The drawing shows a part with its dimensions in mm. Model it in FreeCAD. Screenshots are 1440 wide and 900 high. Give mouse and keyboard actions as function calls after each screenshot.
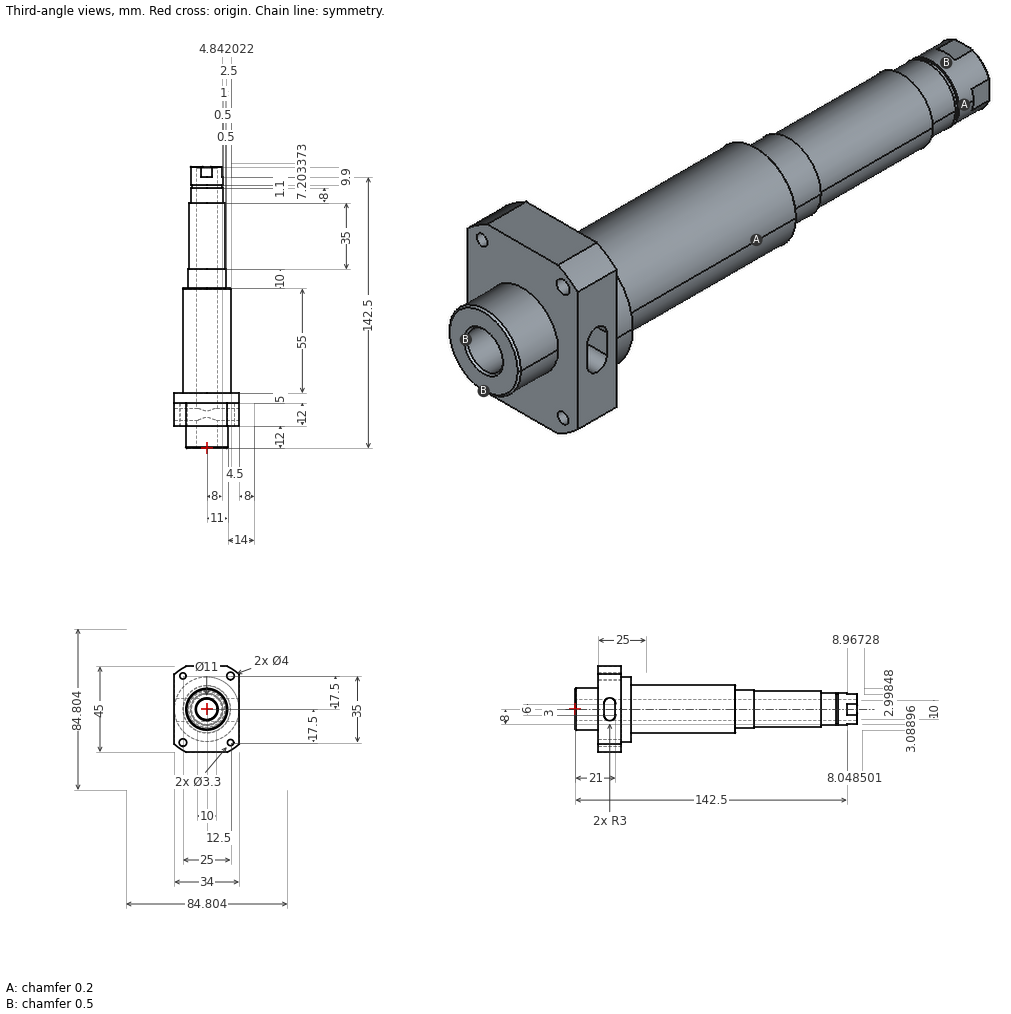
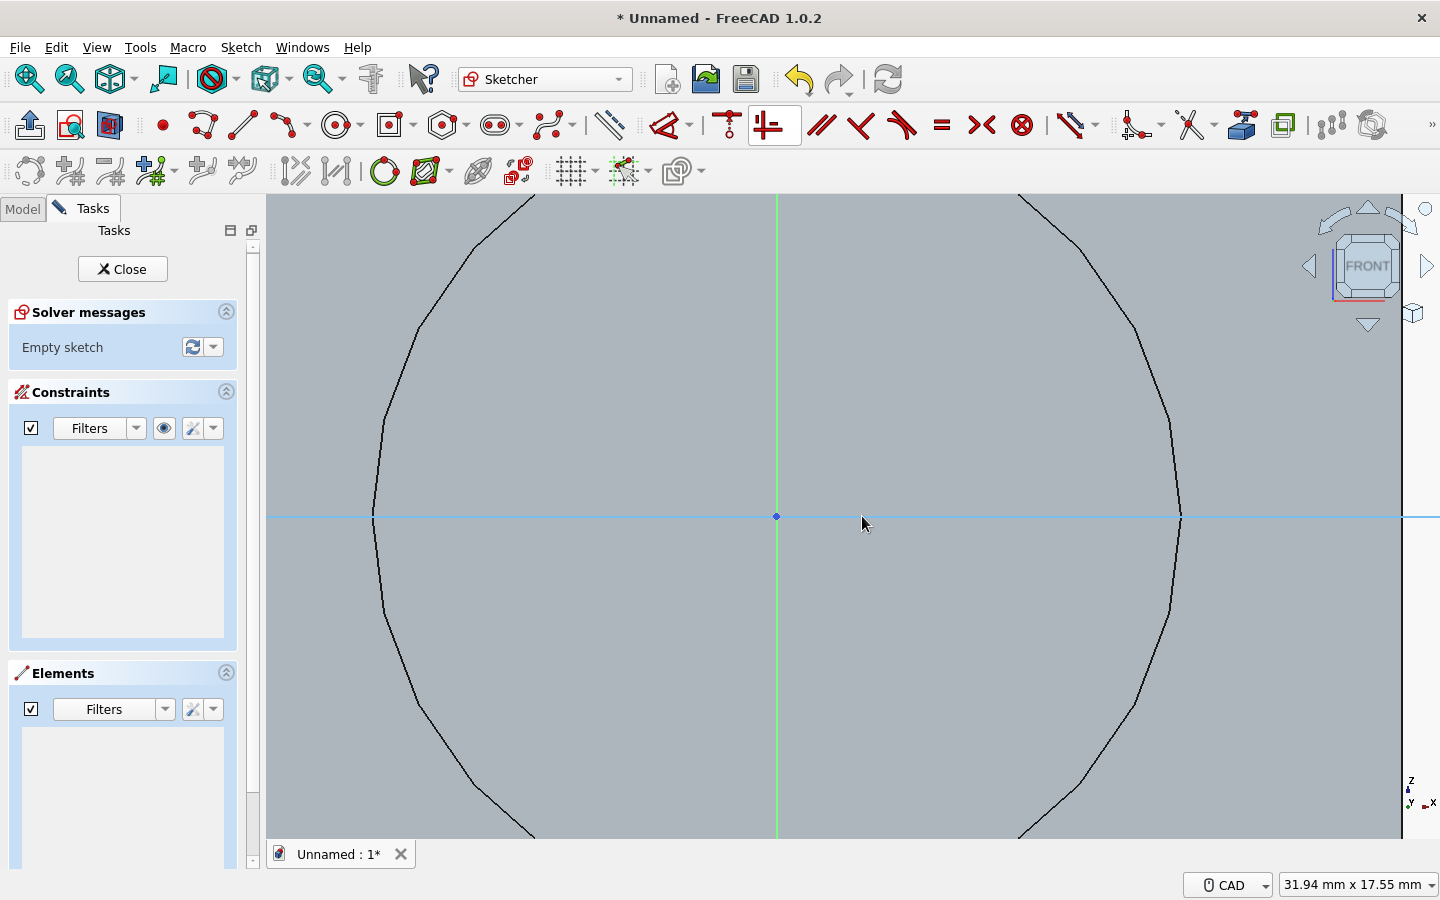
click(336, 126)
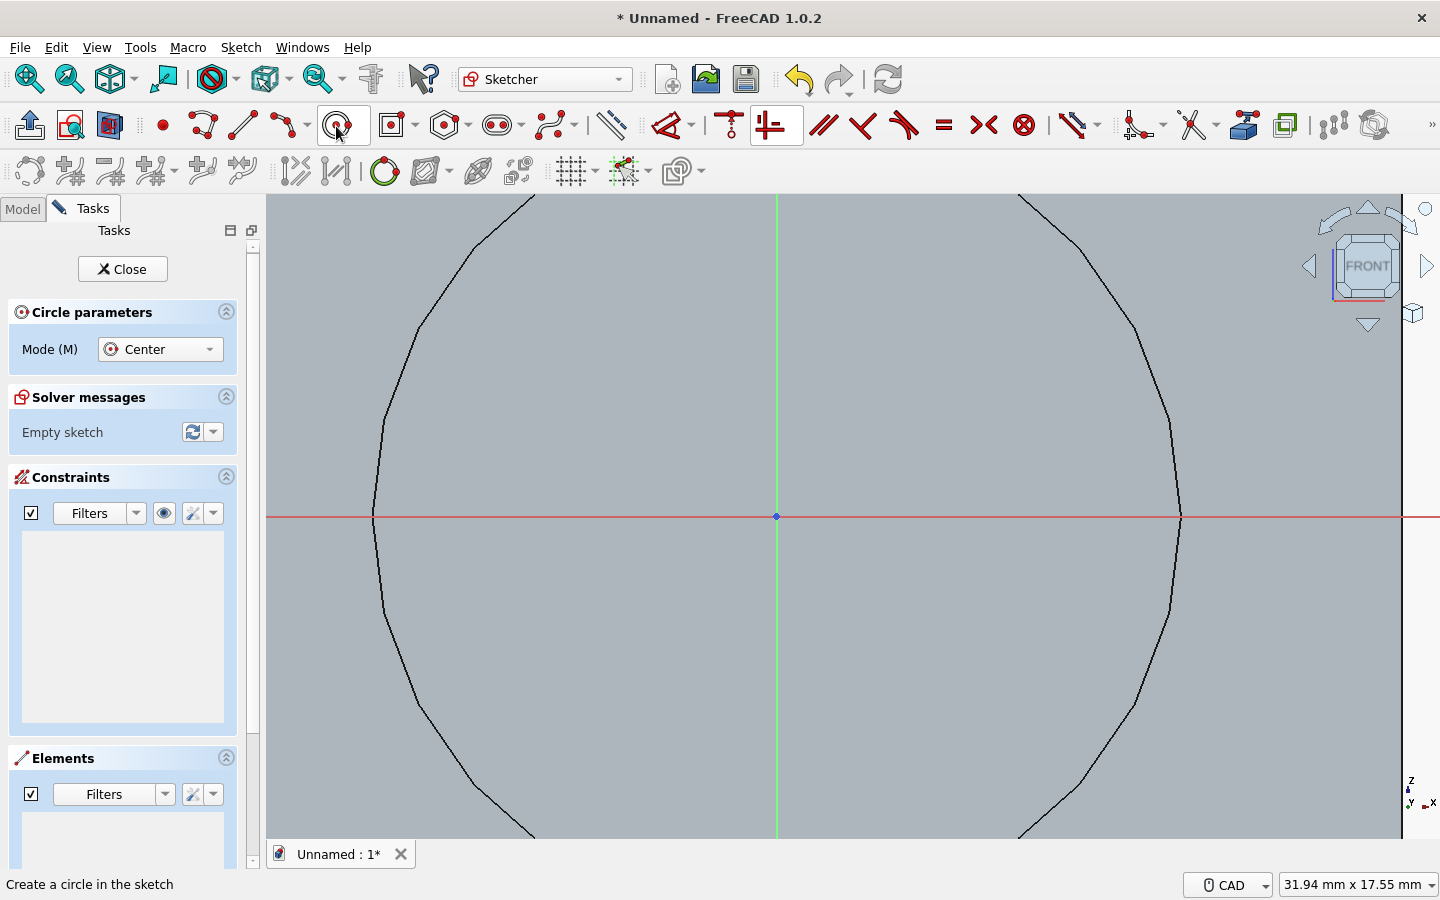
click(777, 516)
move(920, 374)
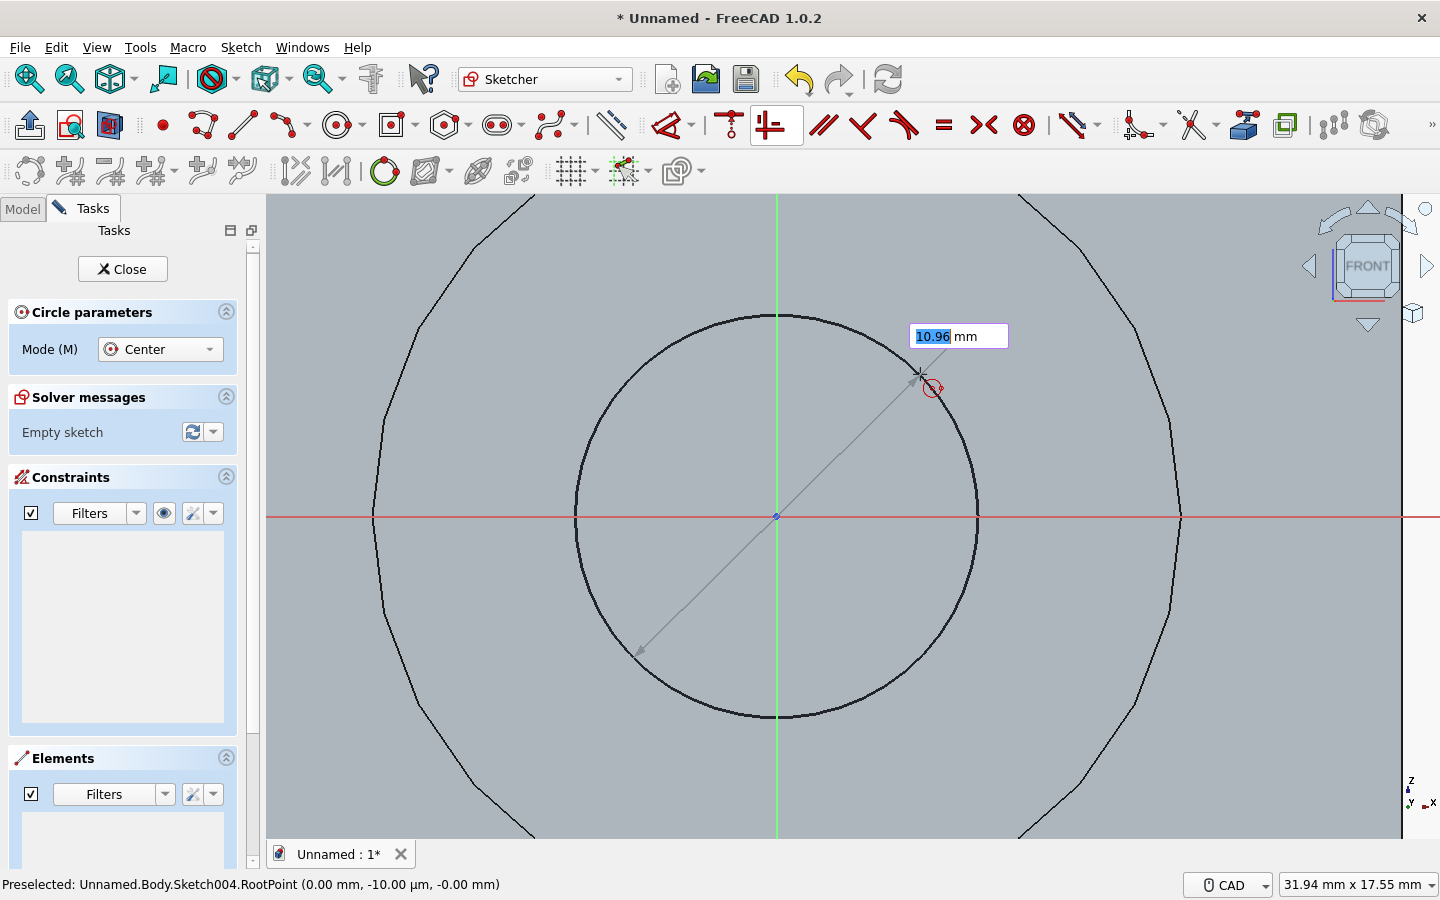
text(11)
key(Return)
key(Escape)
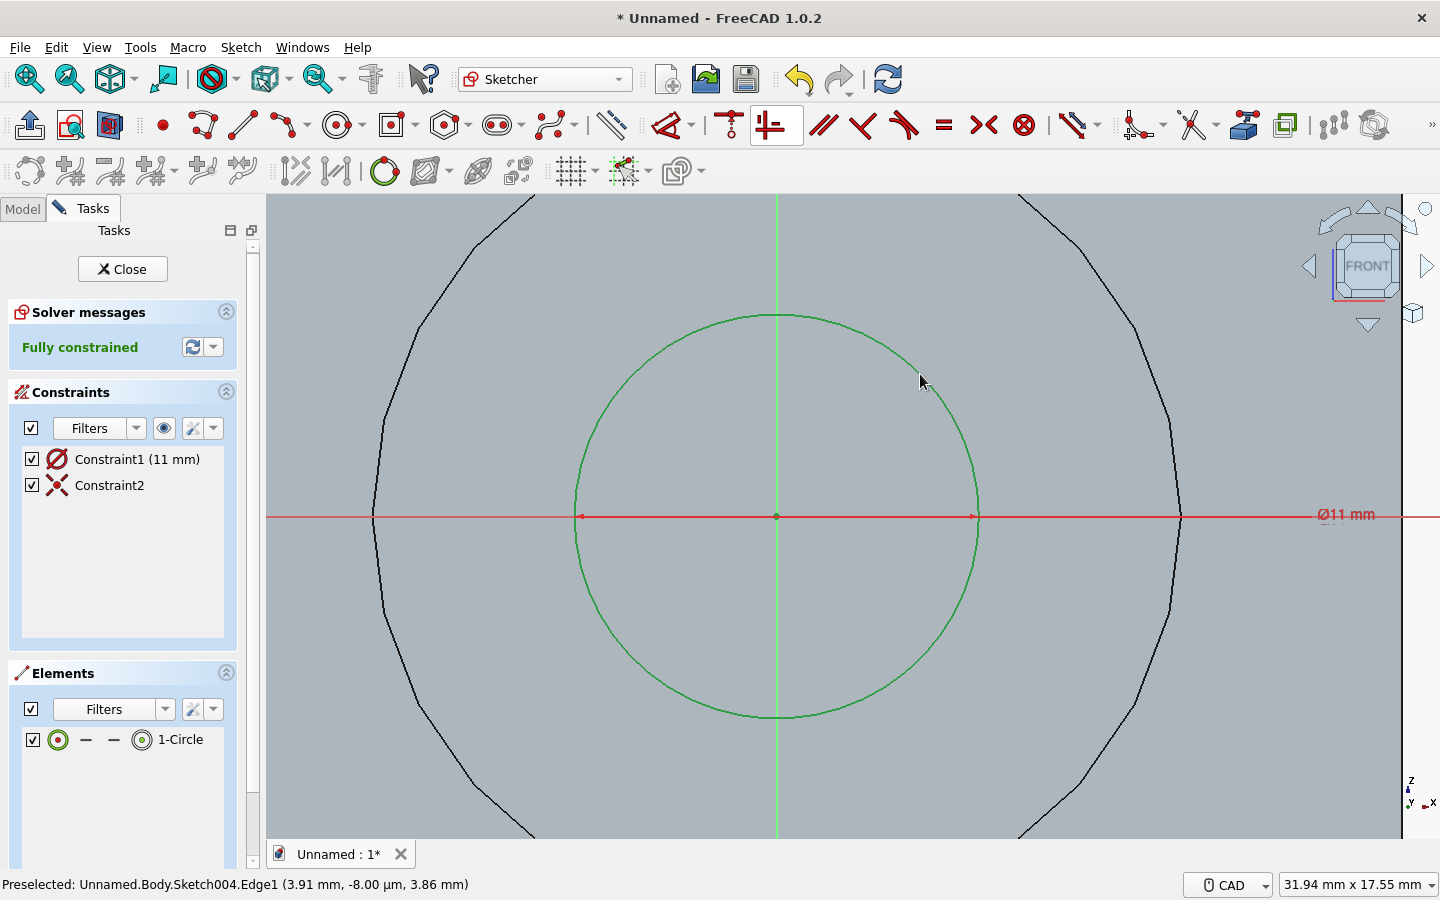
click(123, 269)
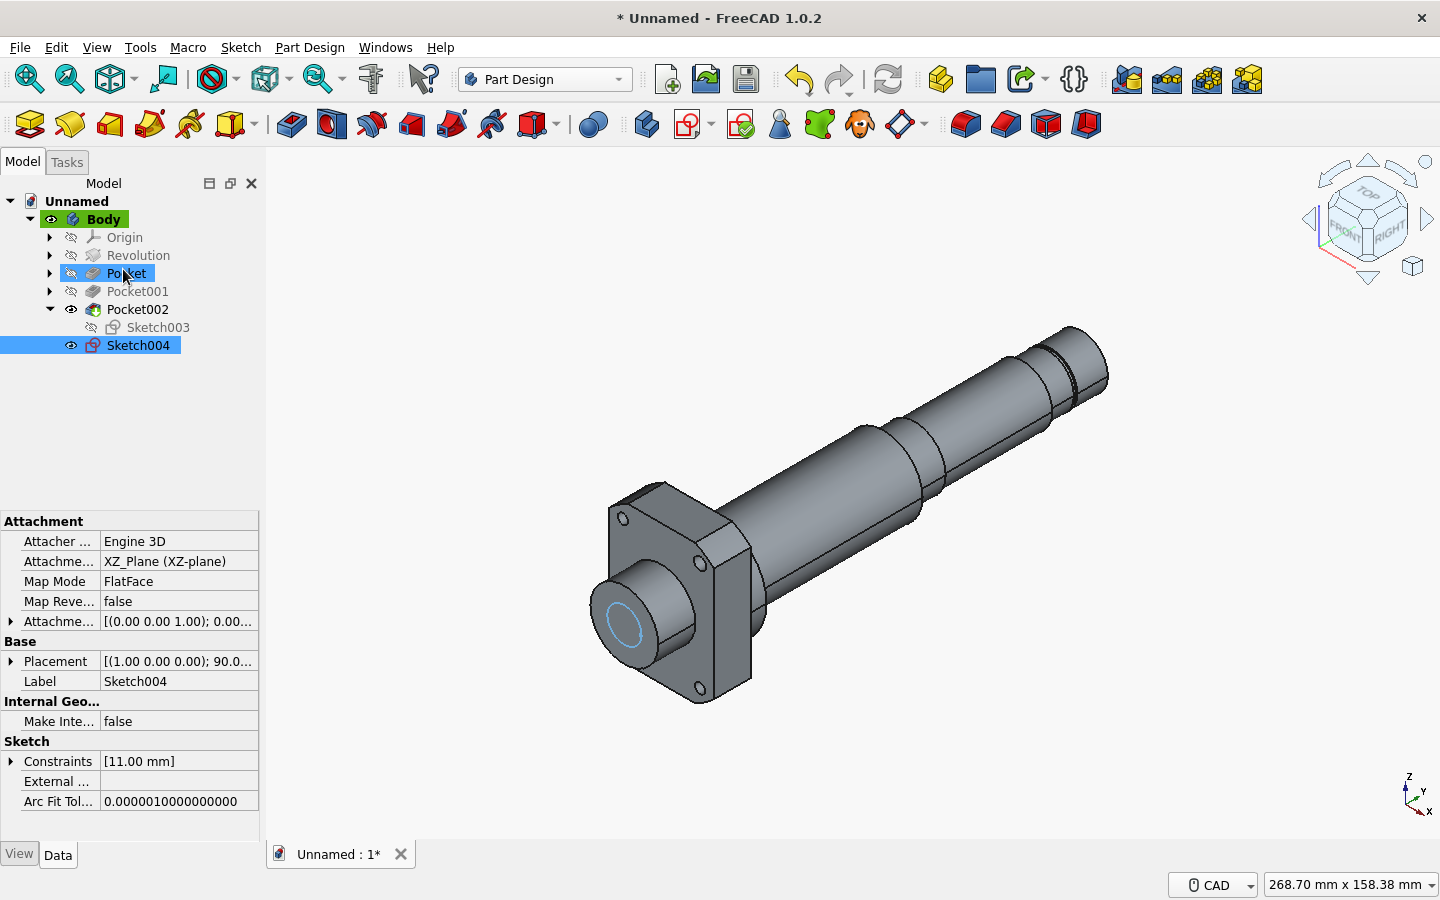
click(292, 124)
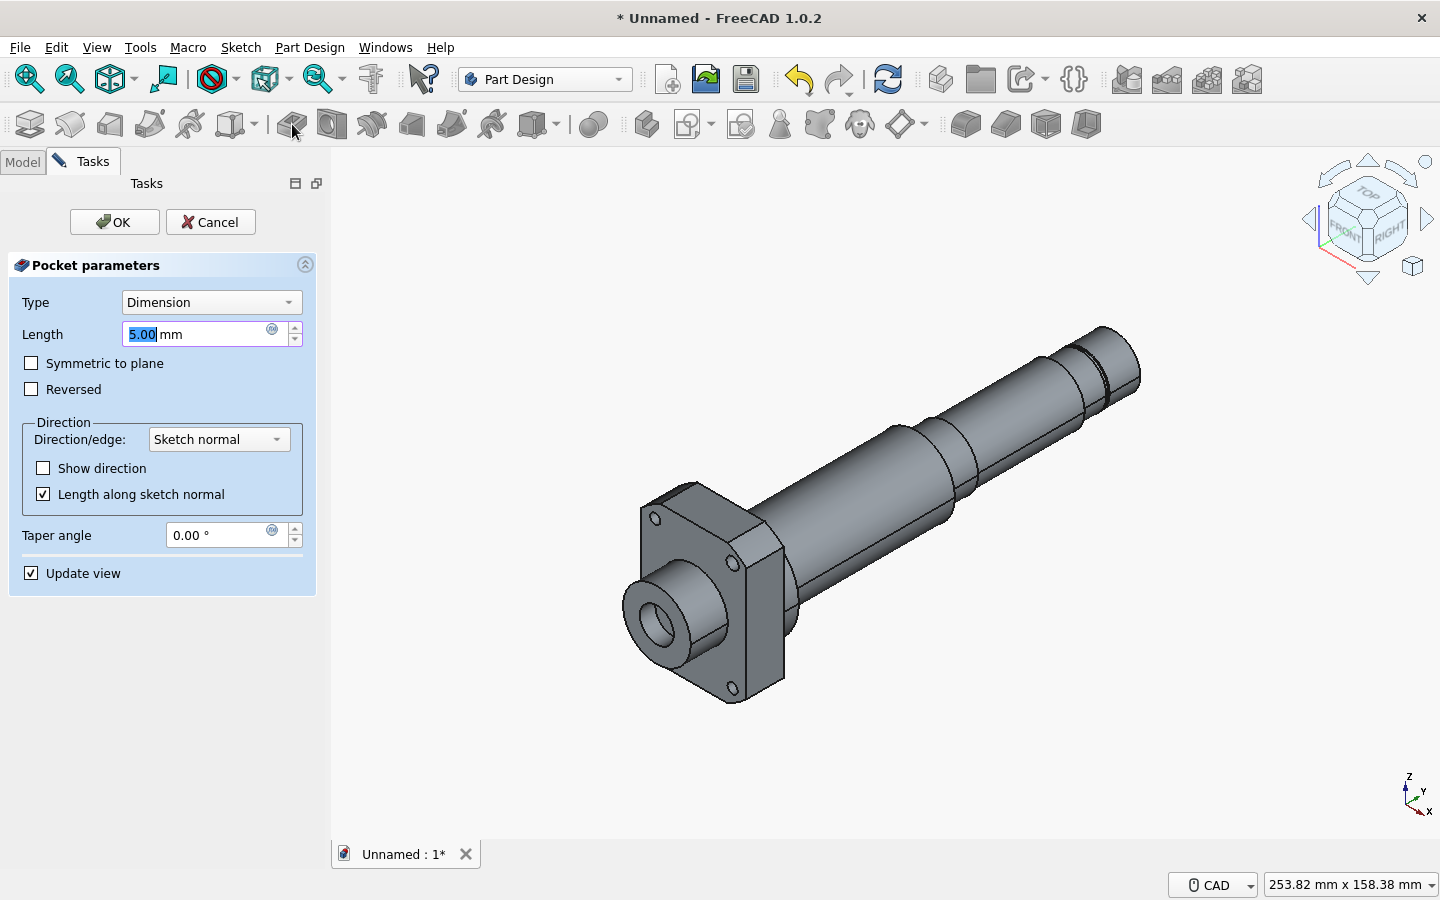
click(212, 302)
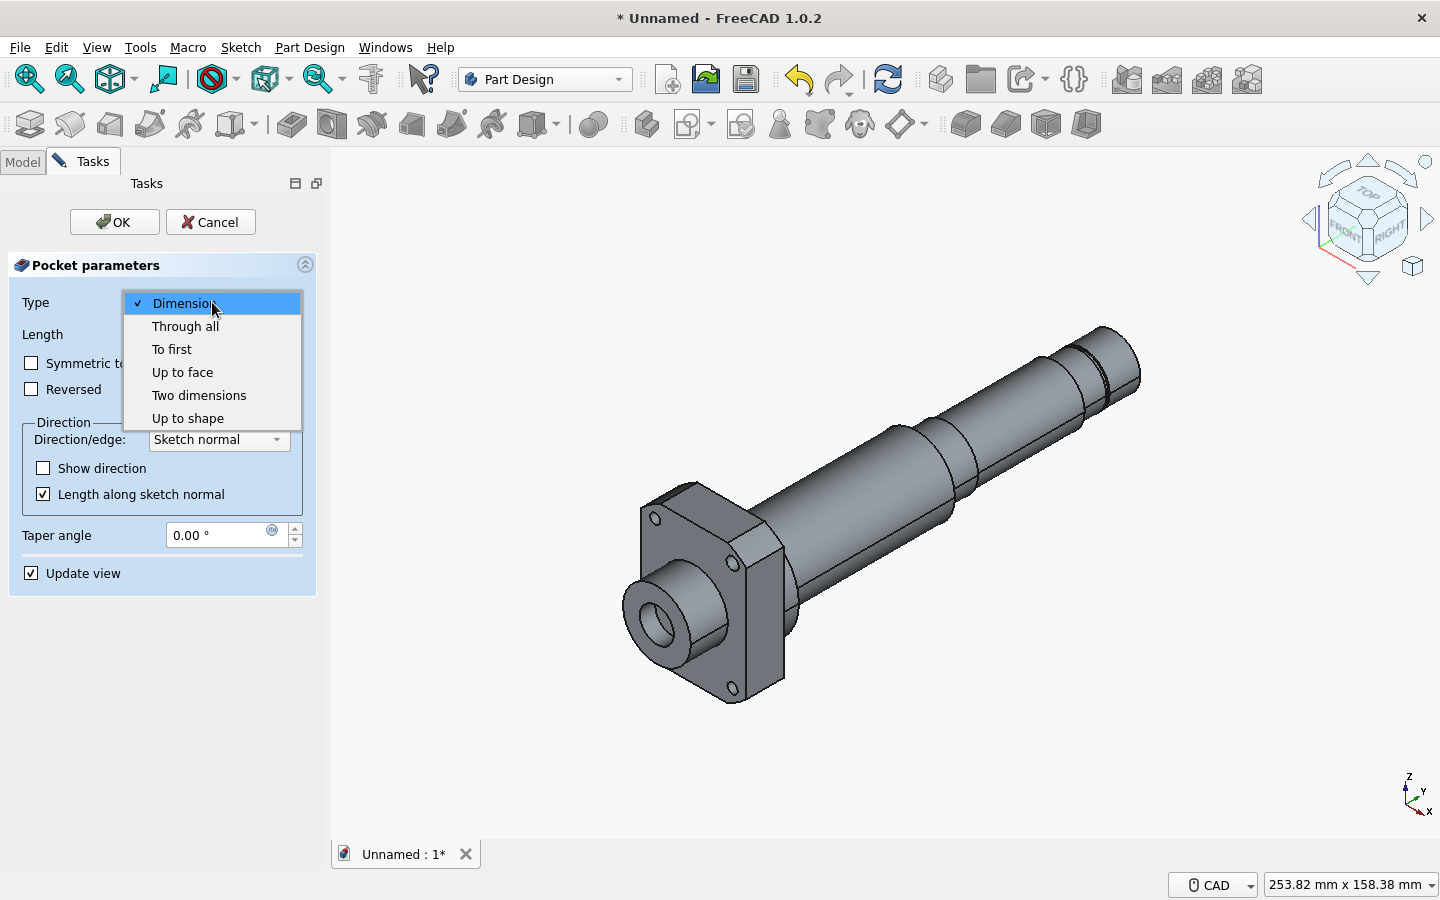
click(212, 326)